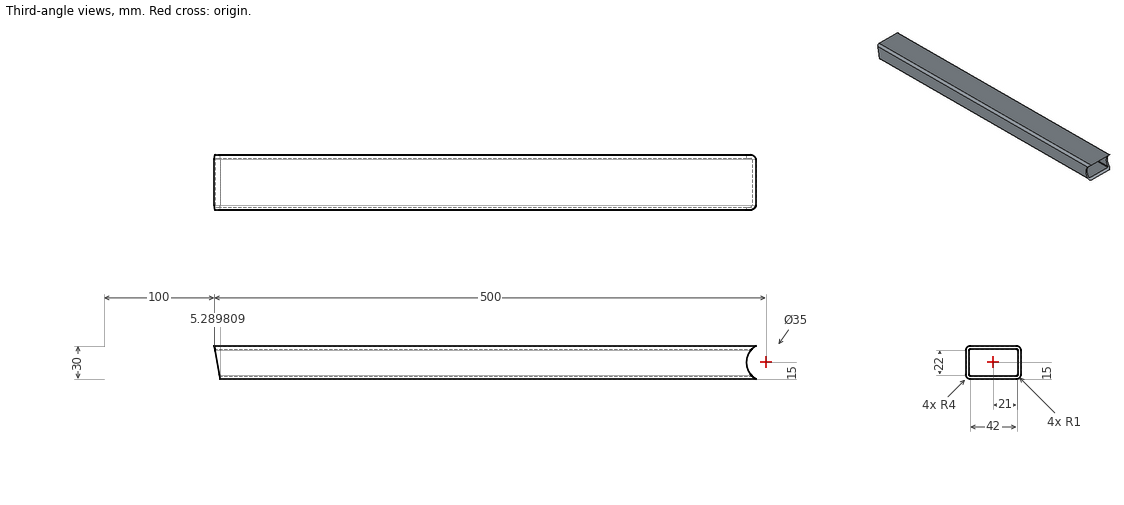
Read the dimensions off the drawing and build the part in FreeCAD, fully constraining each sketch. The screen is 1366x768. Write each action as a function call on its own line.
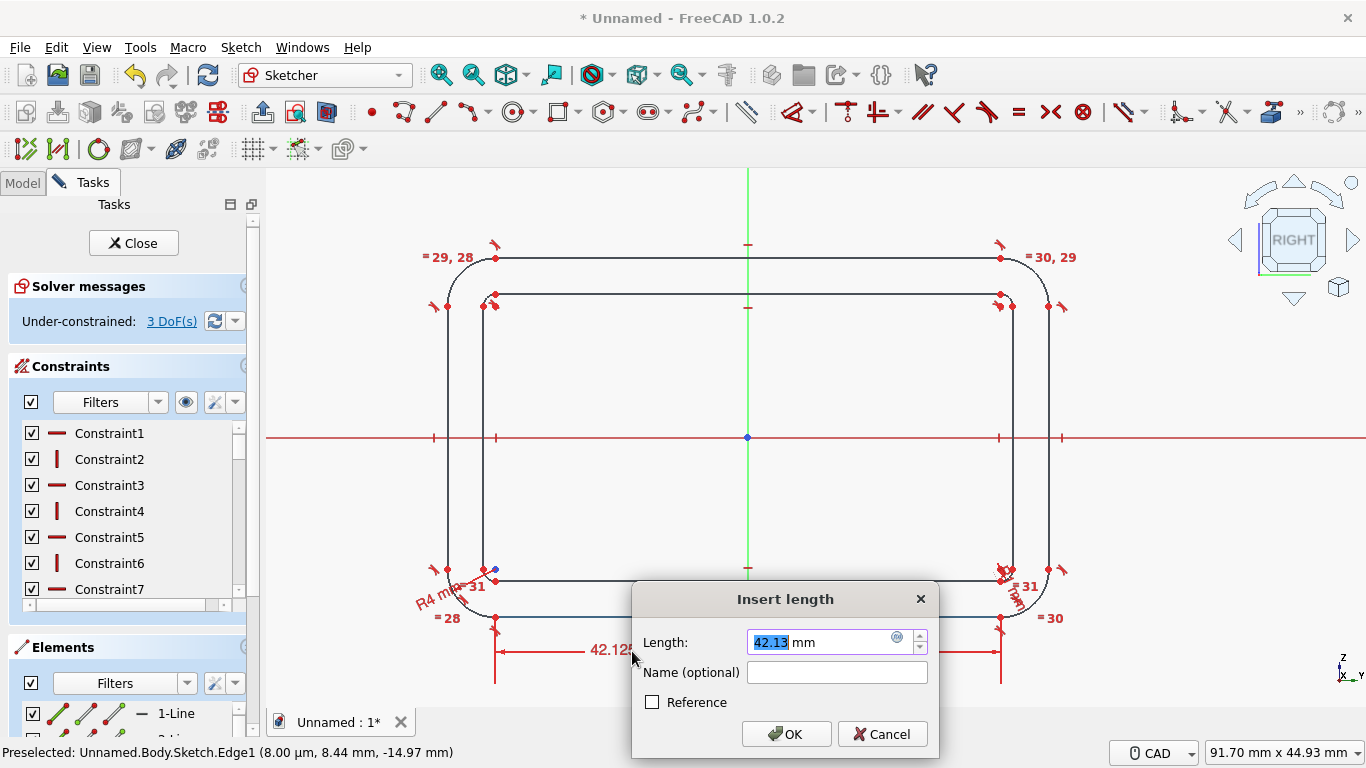
text(42)
key(Return)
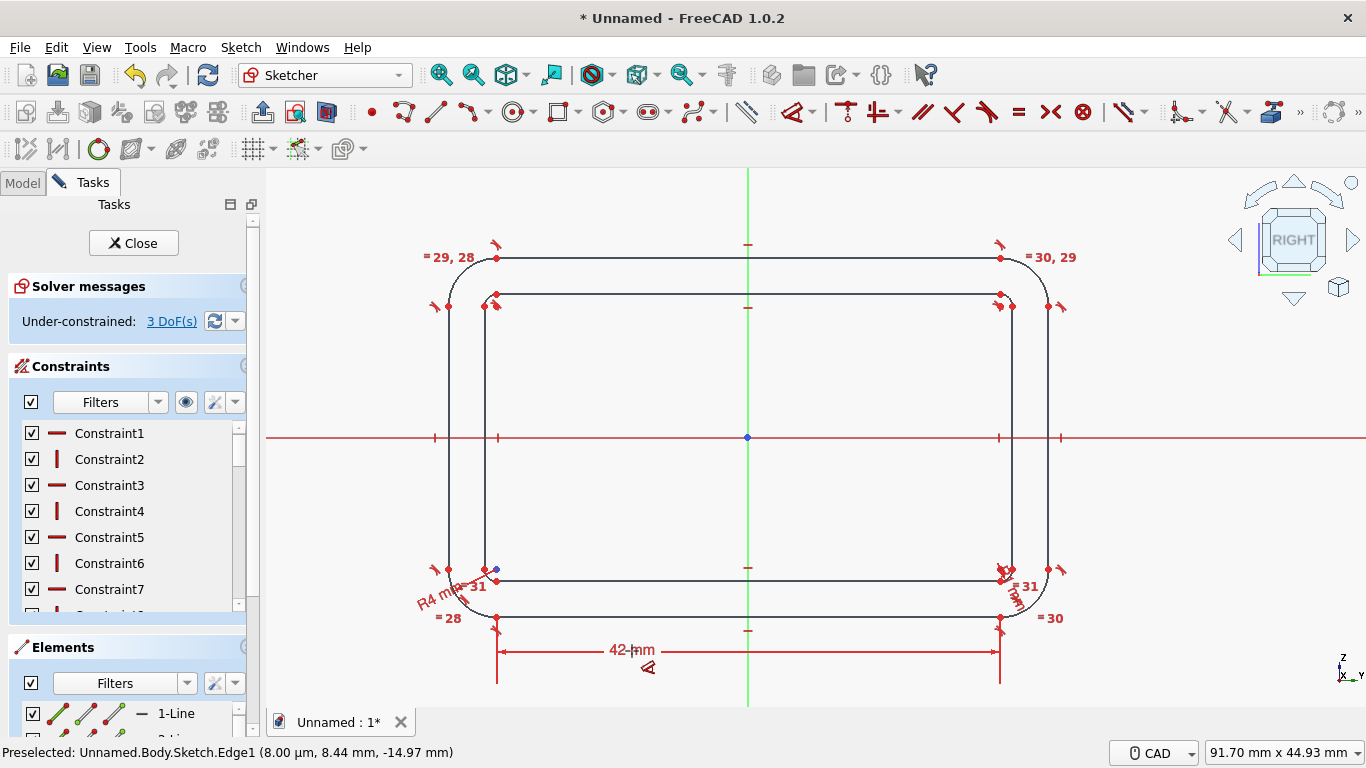
click(449, 490)
click(415, 377)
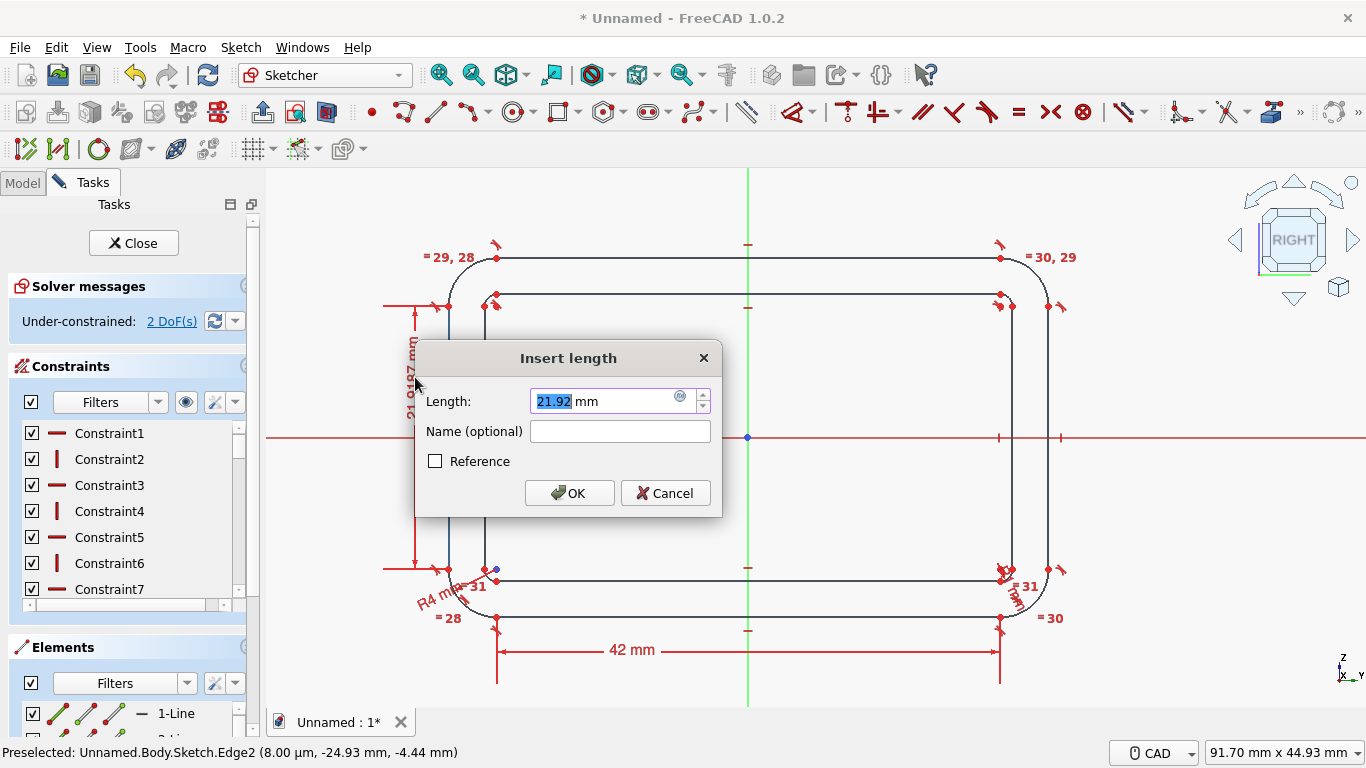
text(22)
key(Return)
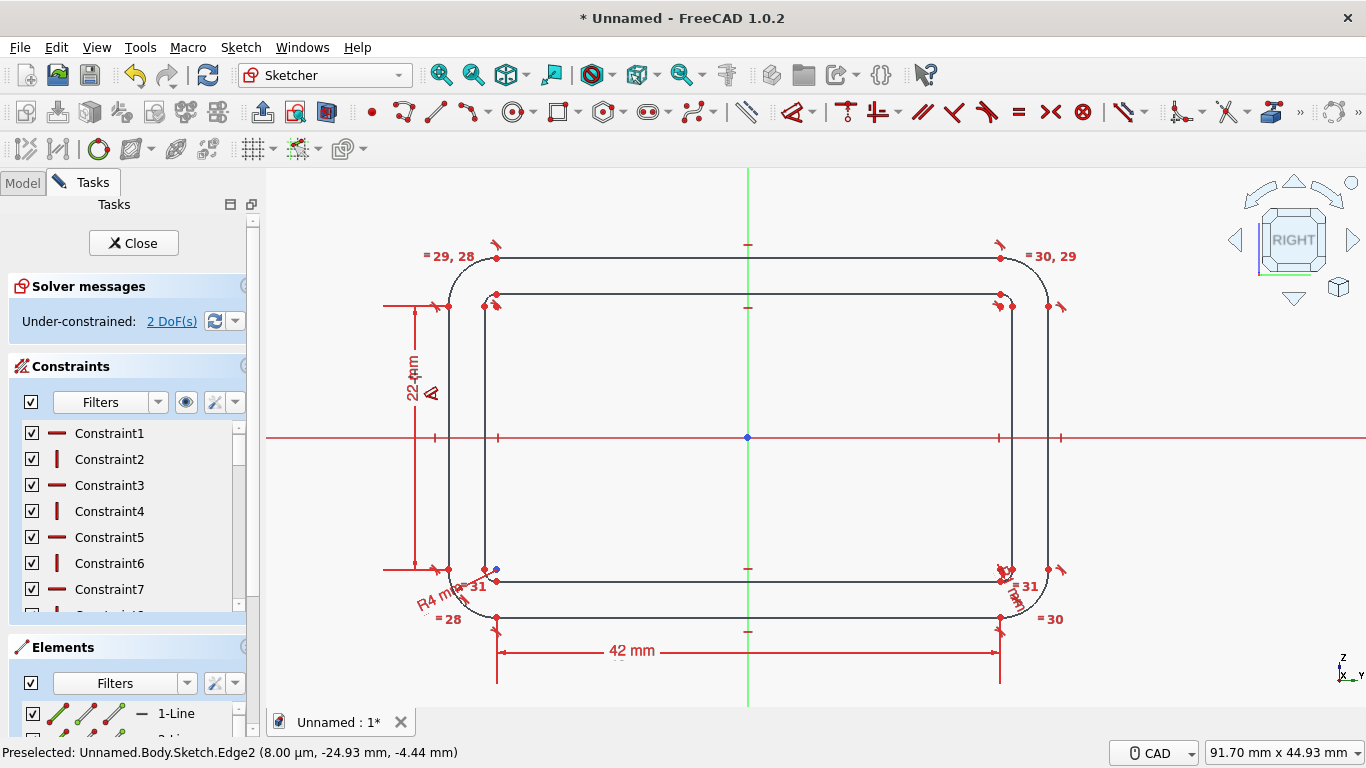
click(1000, 618)
click(874, 652)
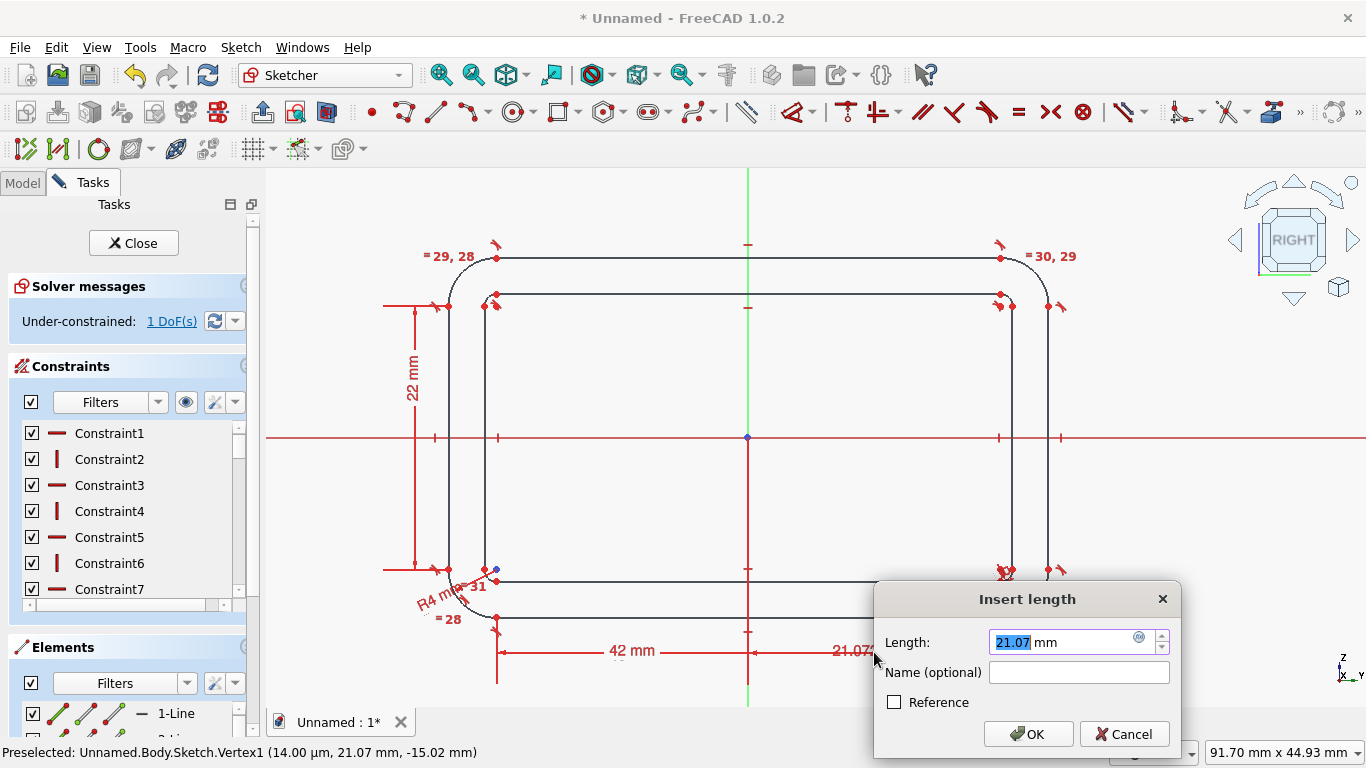
text(21)
key(Return)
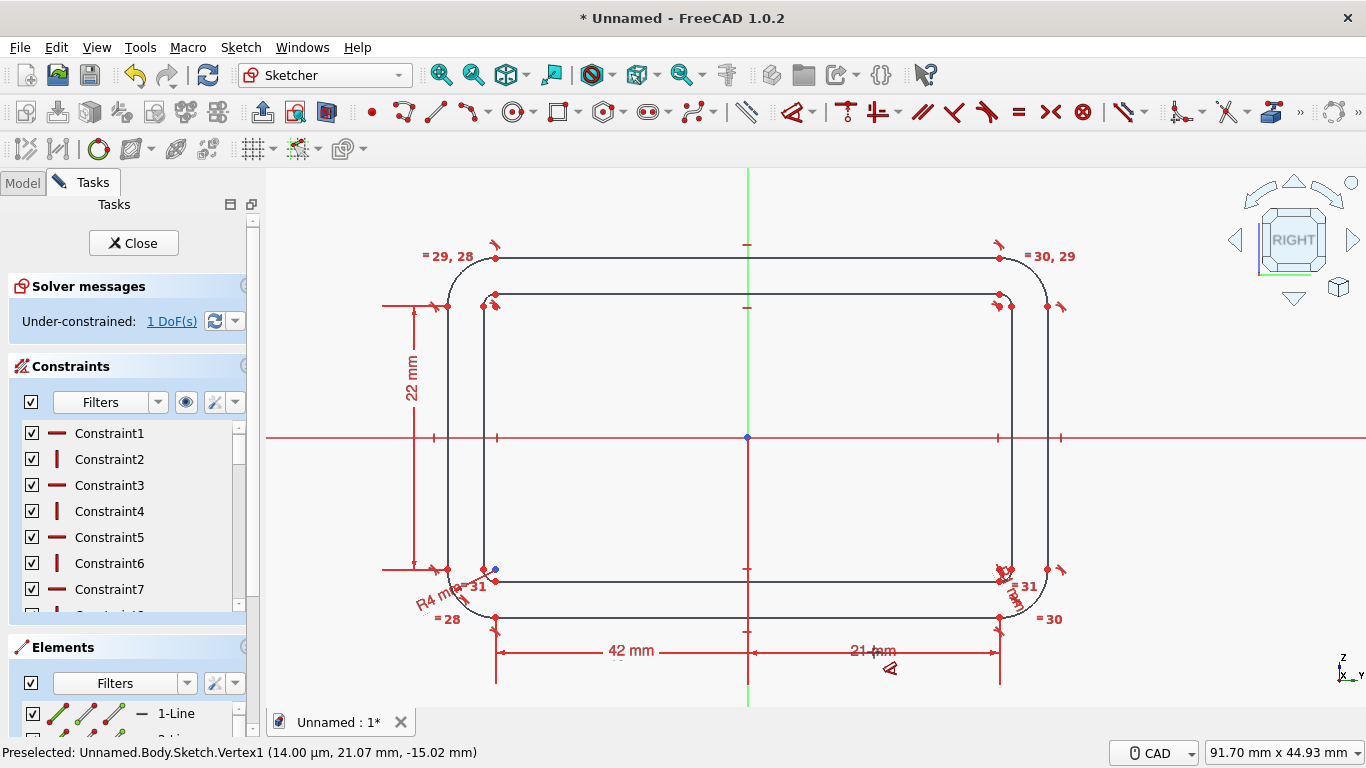
click(1000, 618)
click(1034, 528)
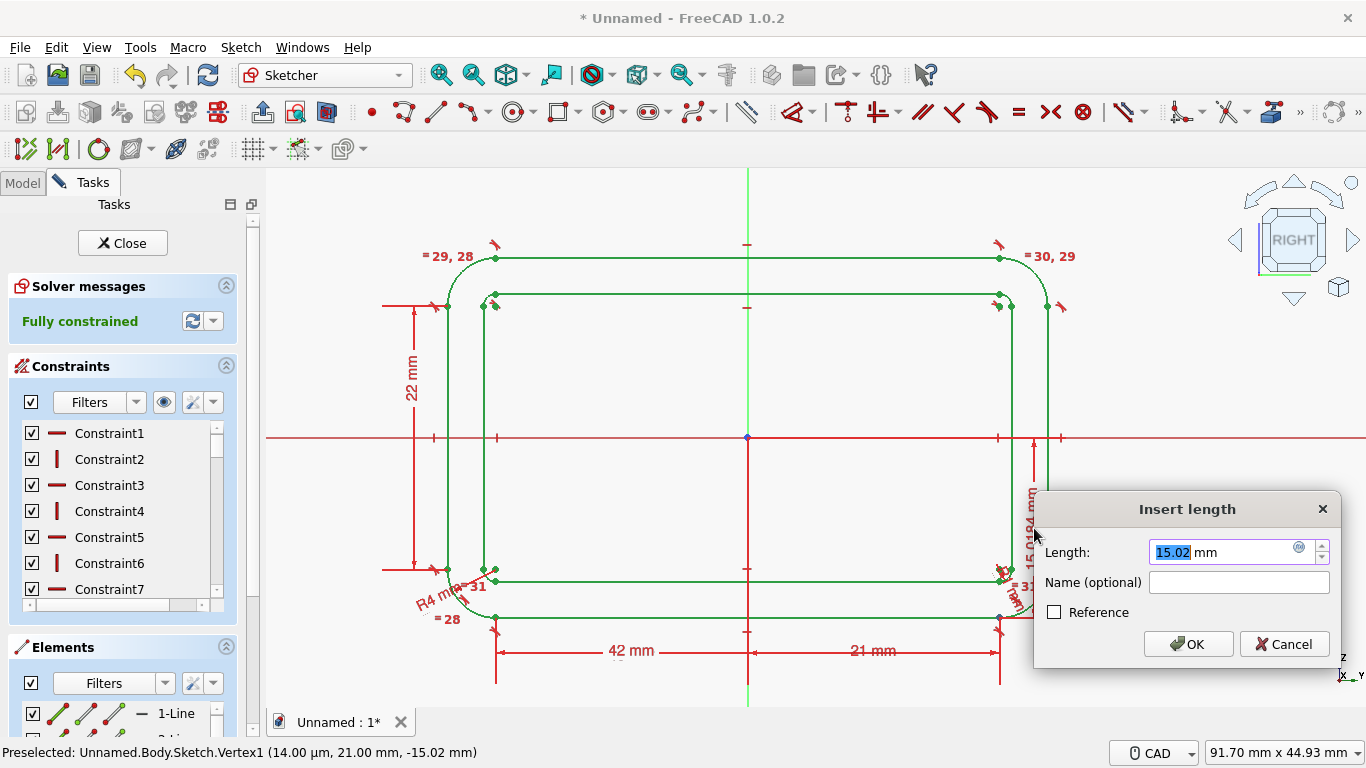
text(15)
key(Return)
key(Escape)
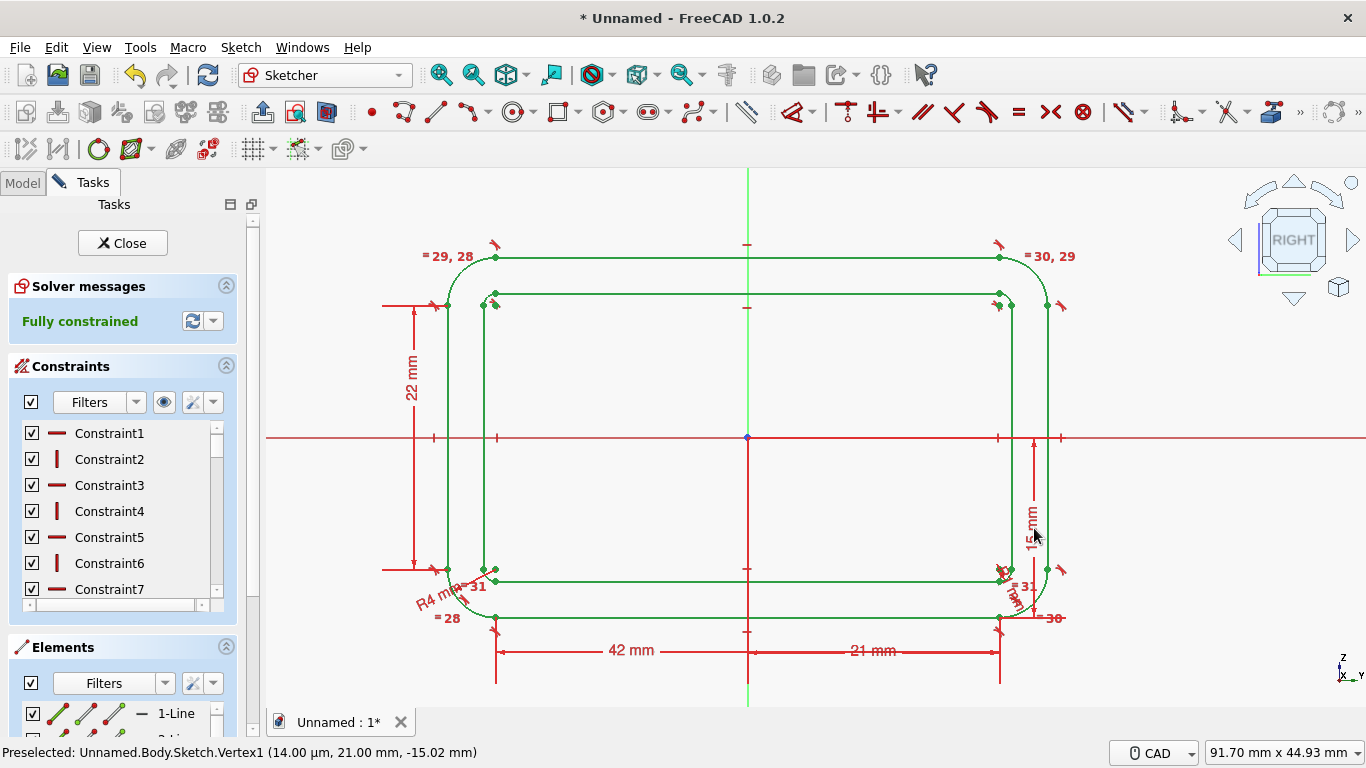
click(123, 243)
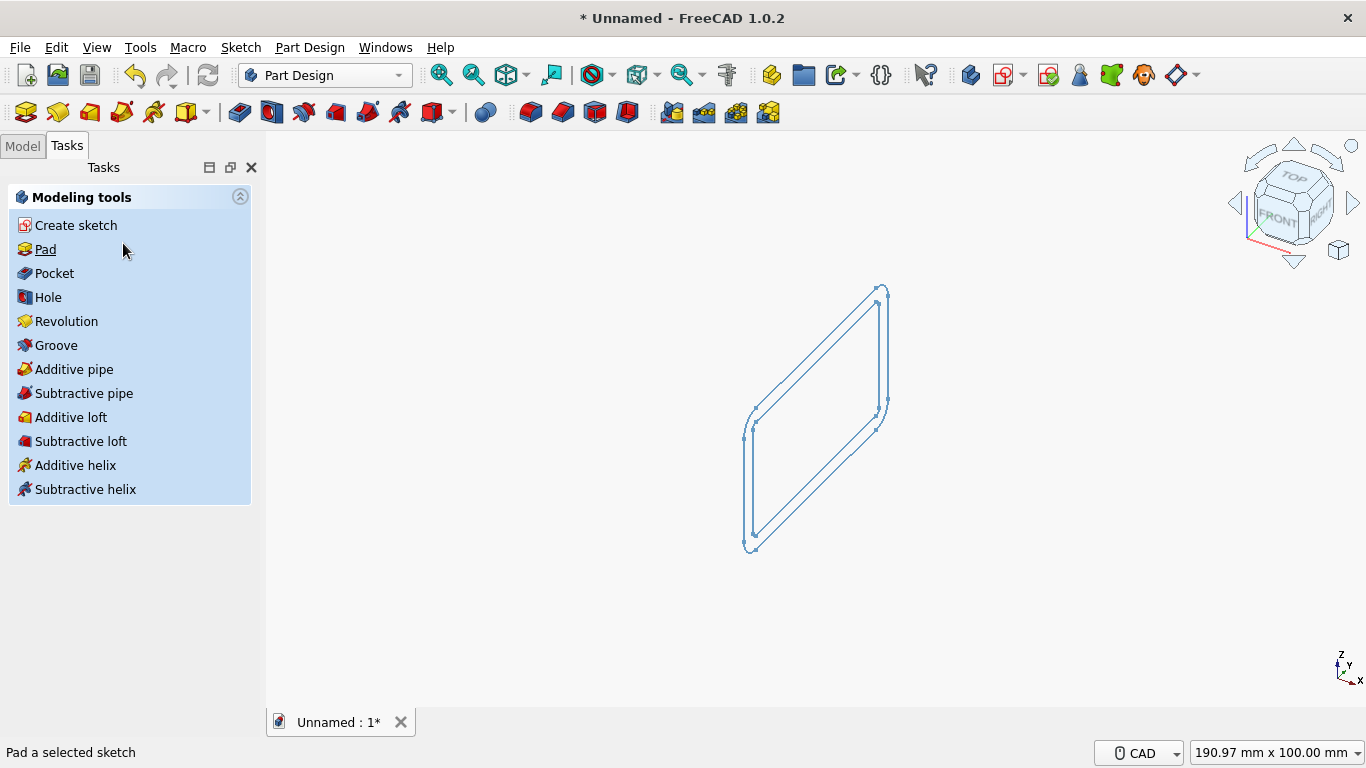
click(26, 112)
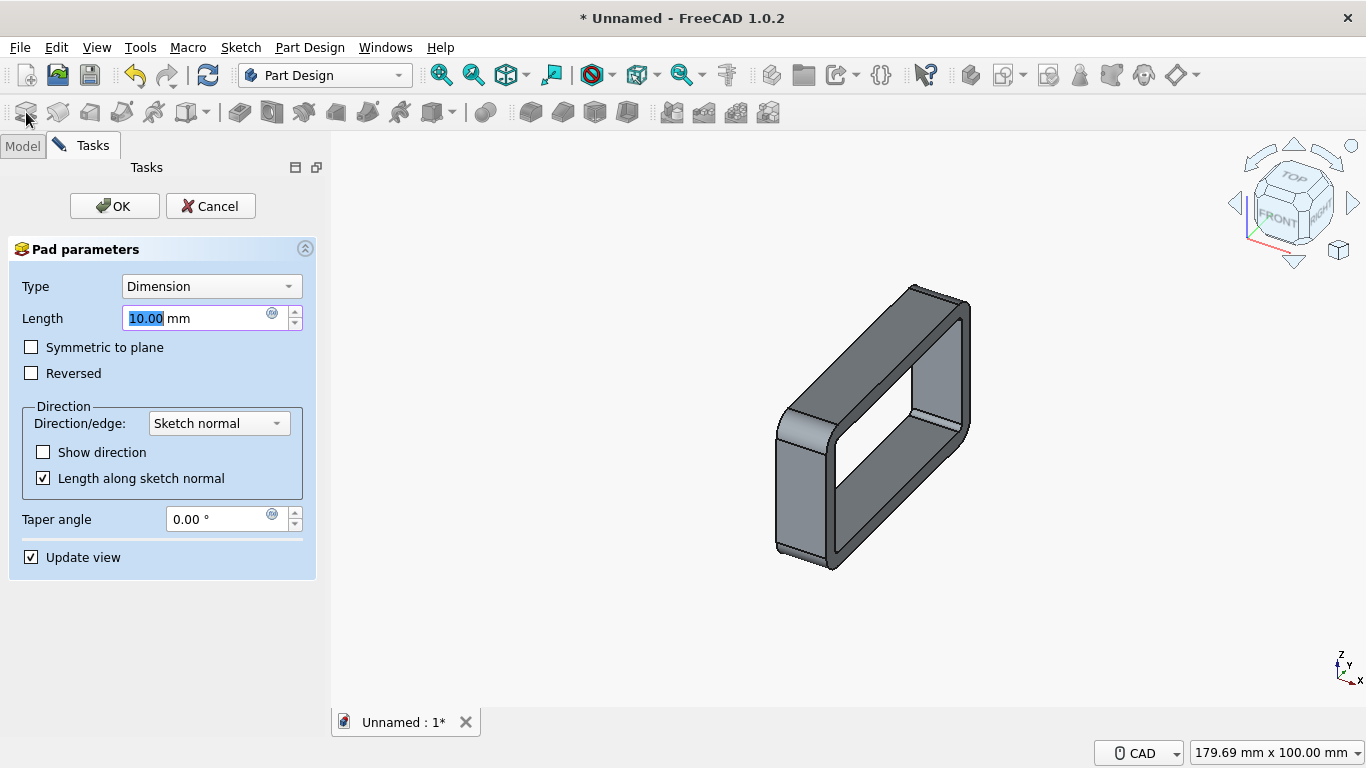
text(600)
key(Tab)